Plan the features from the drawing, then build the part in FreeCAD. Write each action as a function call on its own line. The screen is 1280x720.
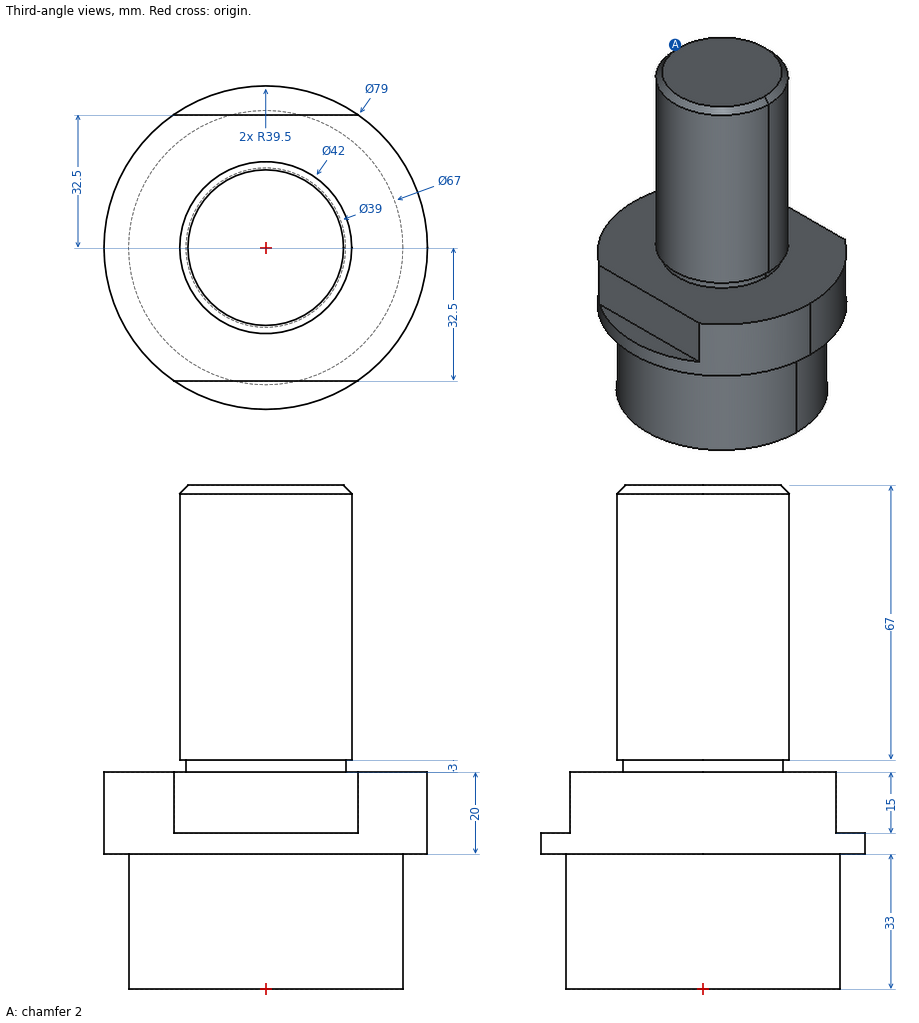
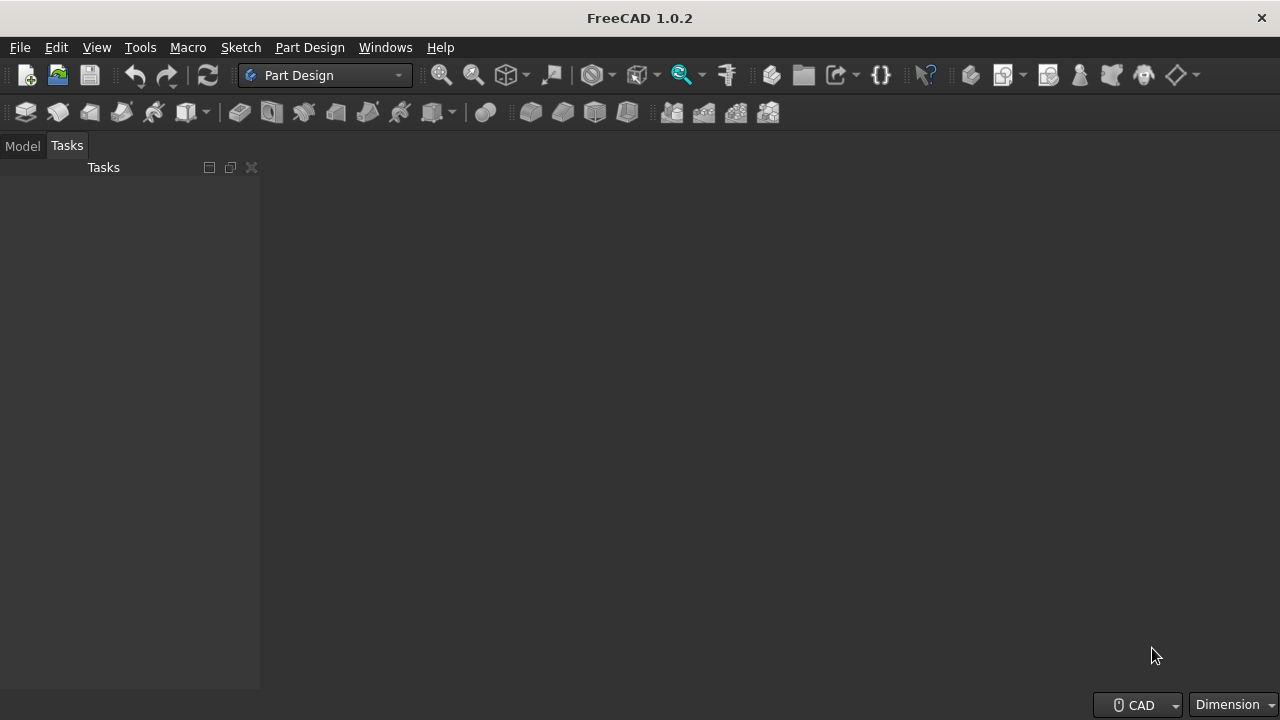
click(26, 76)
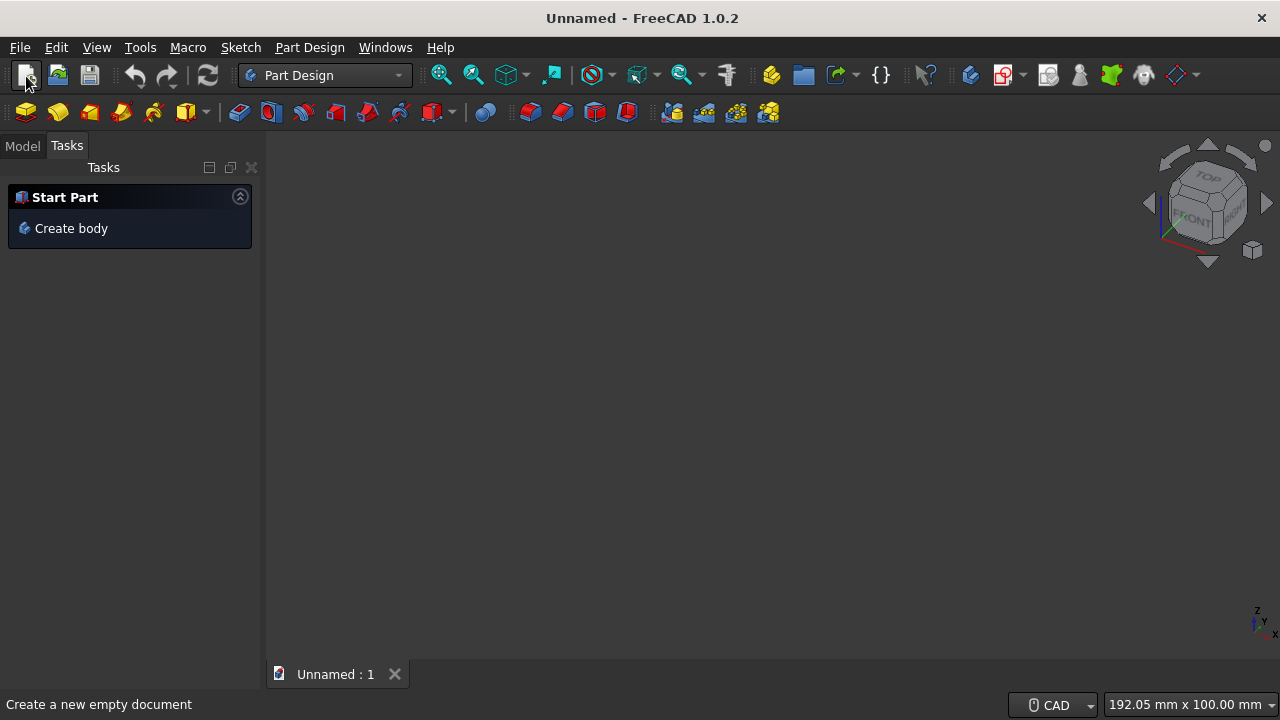
click(1004, 76)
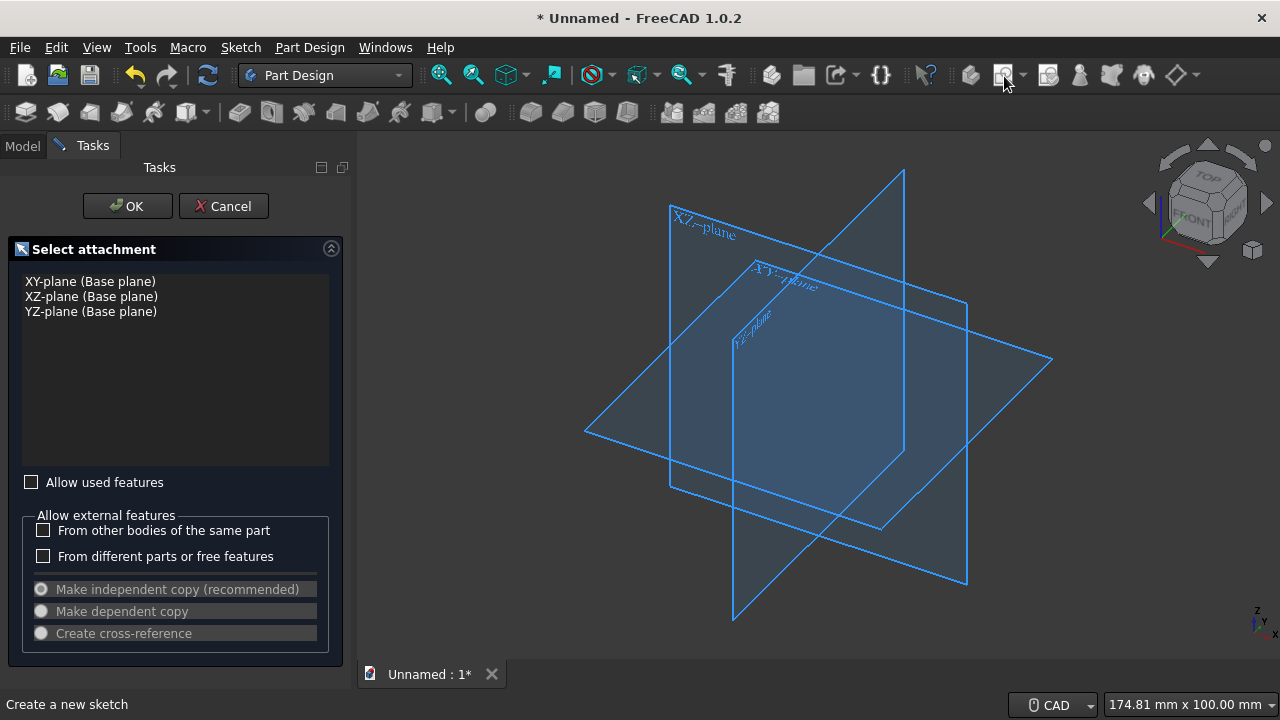
click(82, 282)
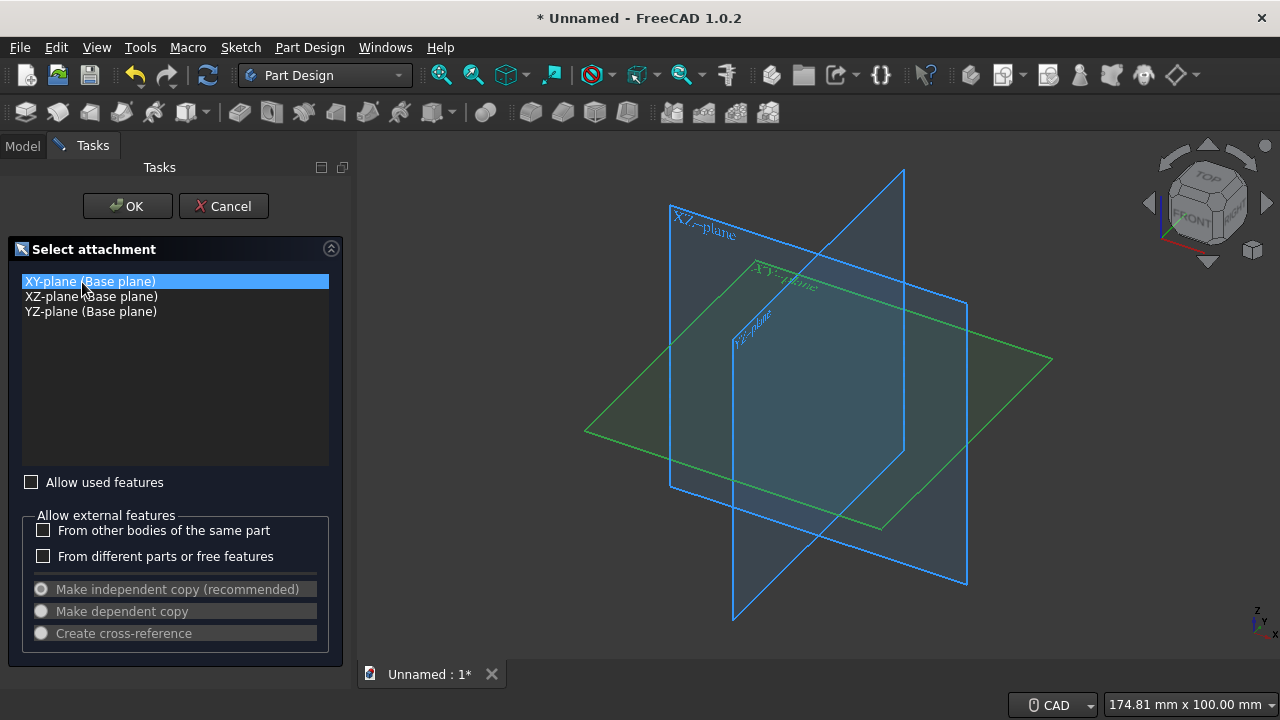
click(128, 206)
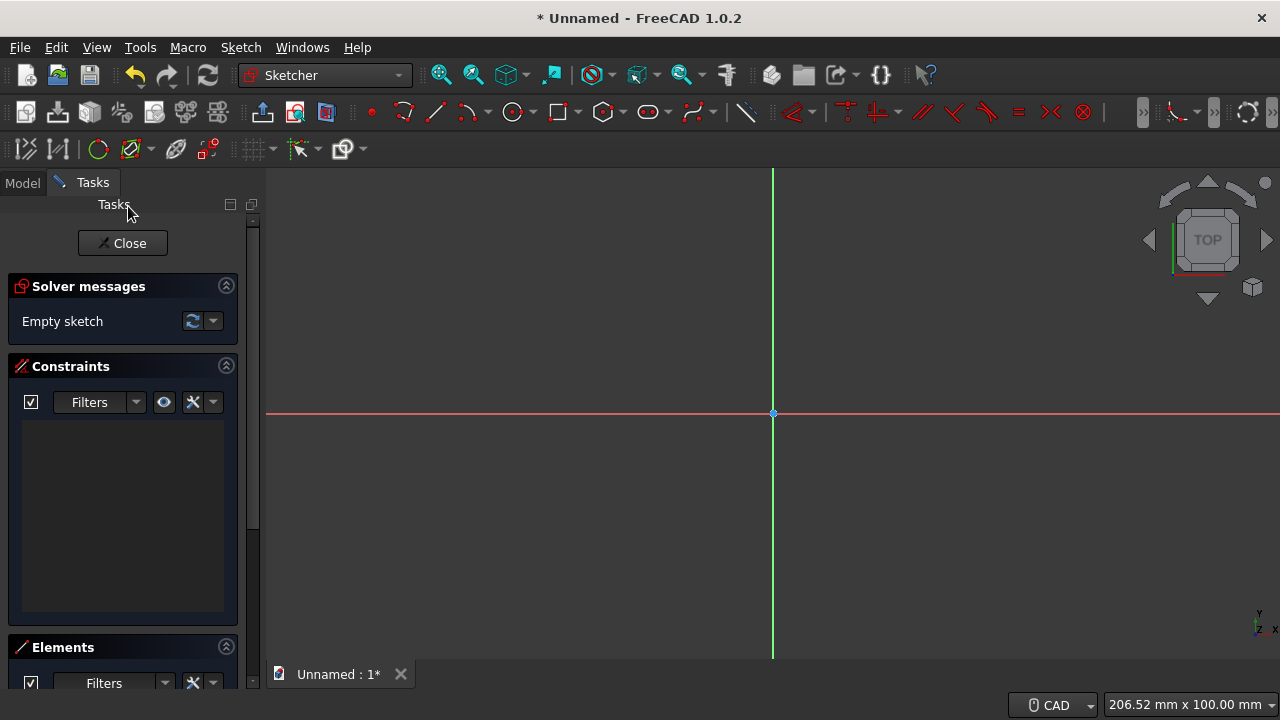
click(514, 112)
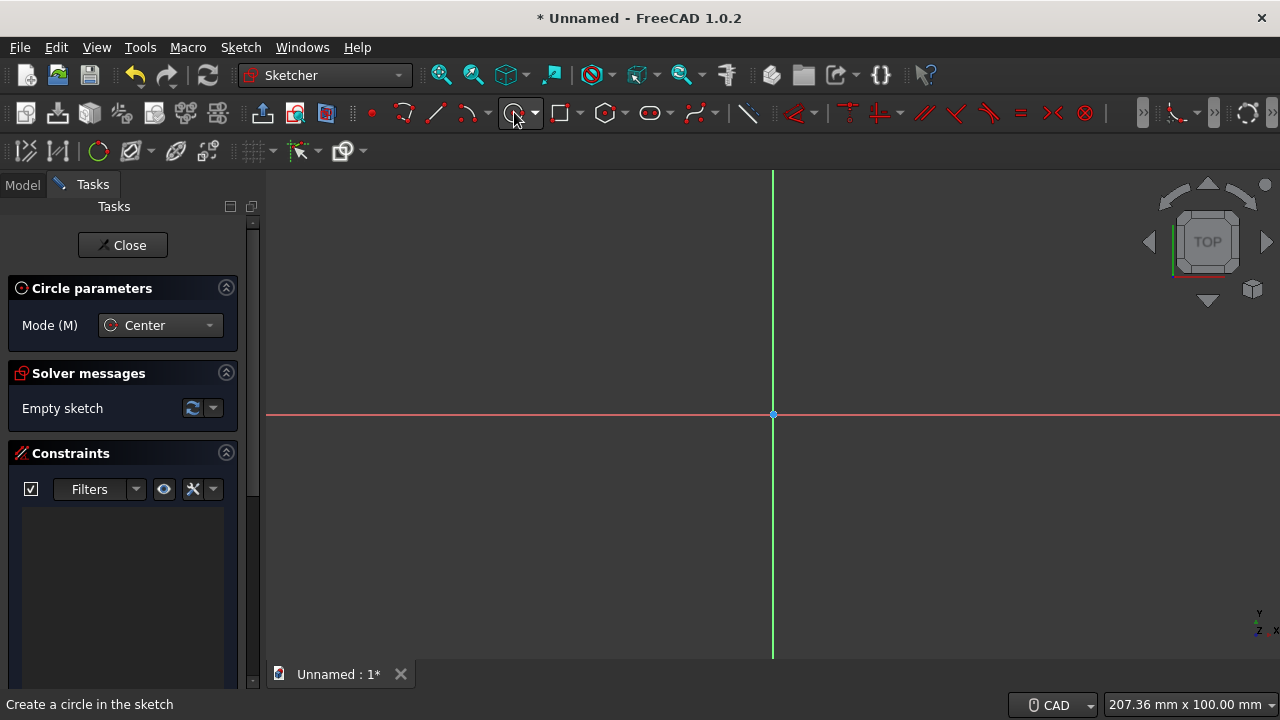
click(773, 414)
move(889, 299)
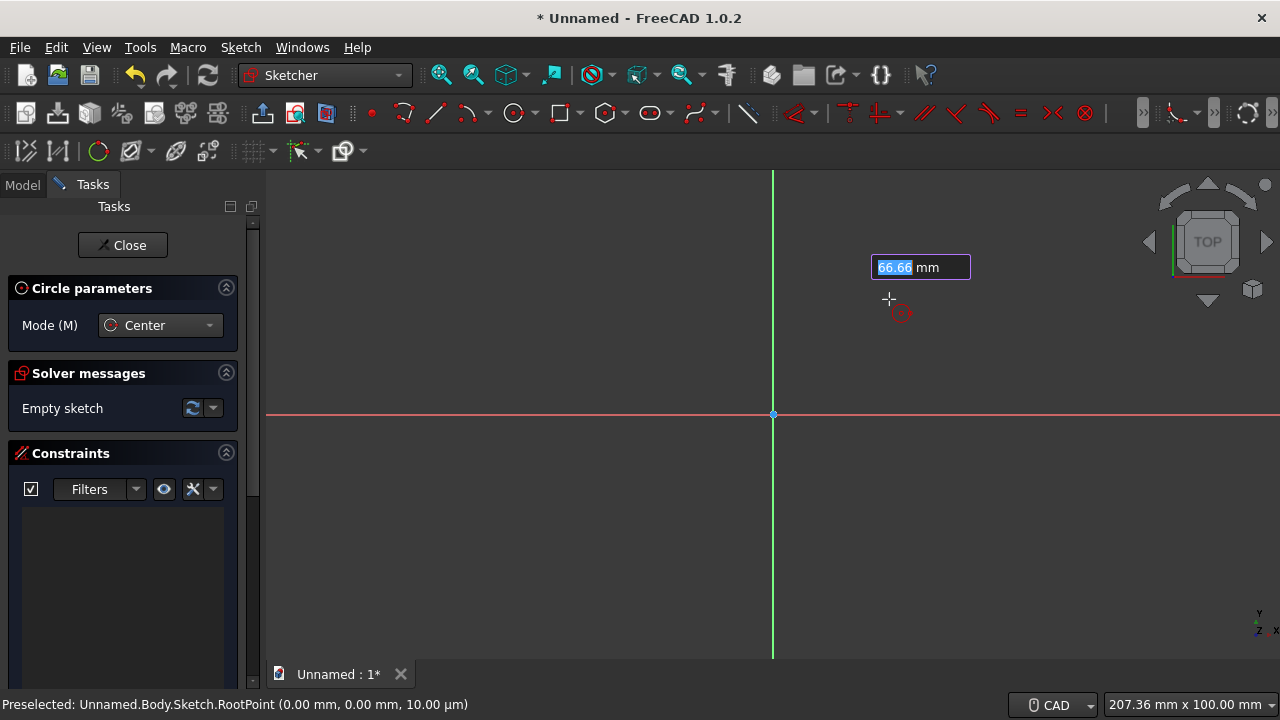
text(67)
key(Return)
key(Escape)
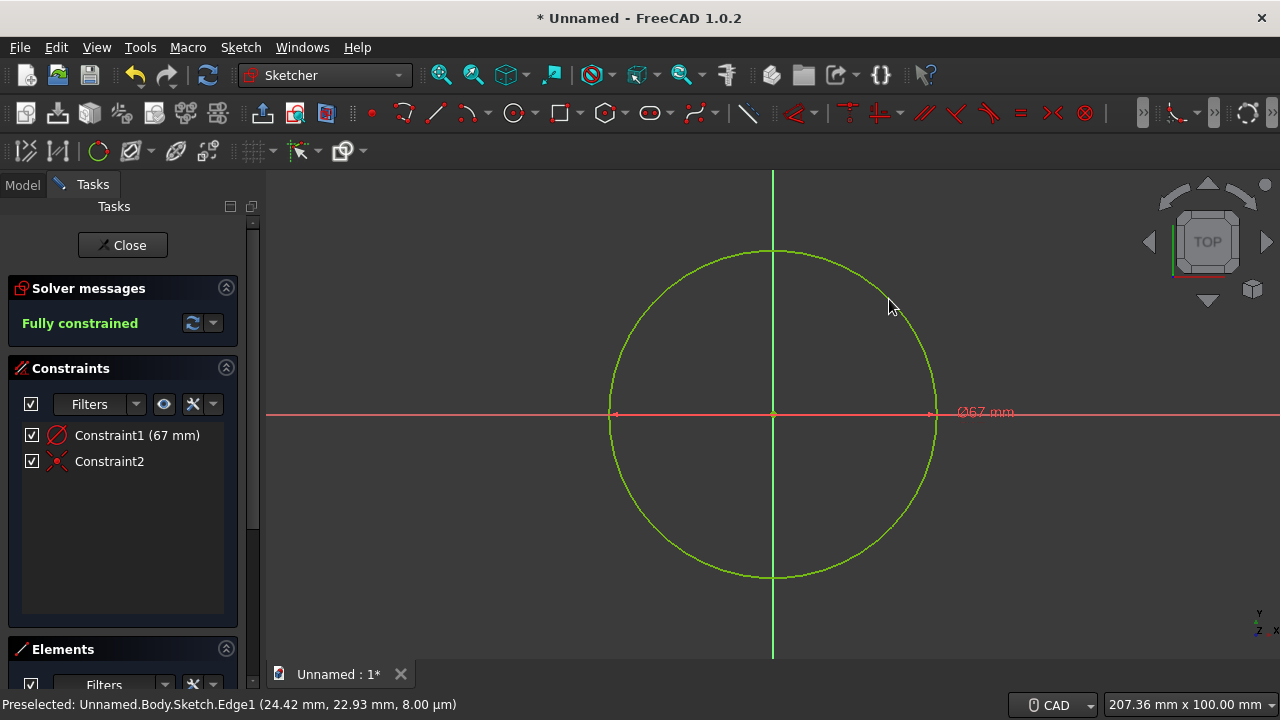
click(123, 245)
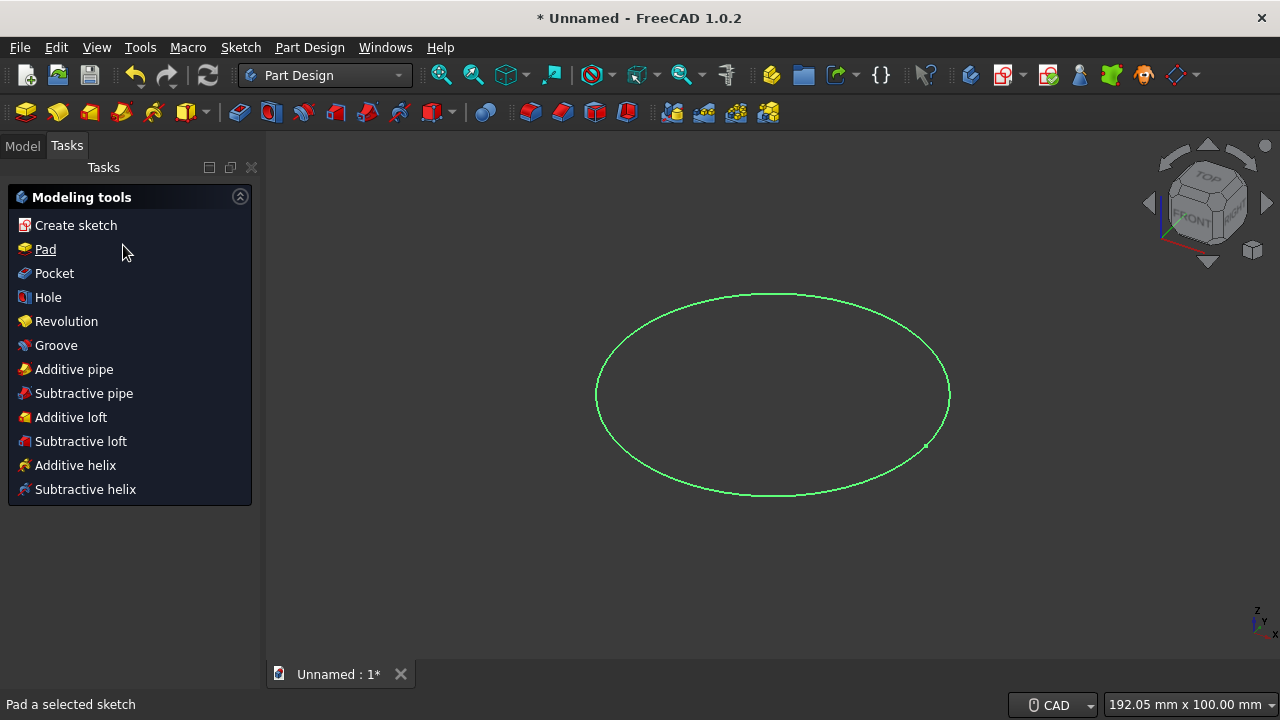
click(26, 112)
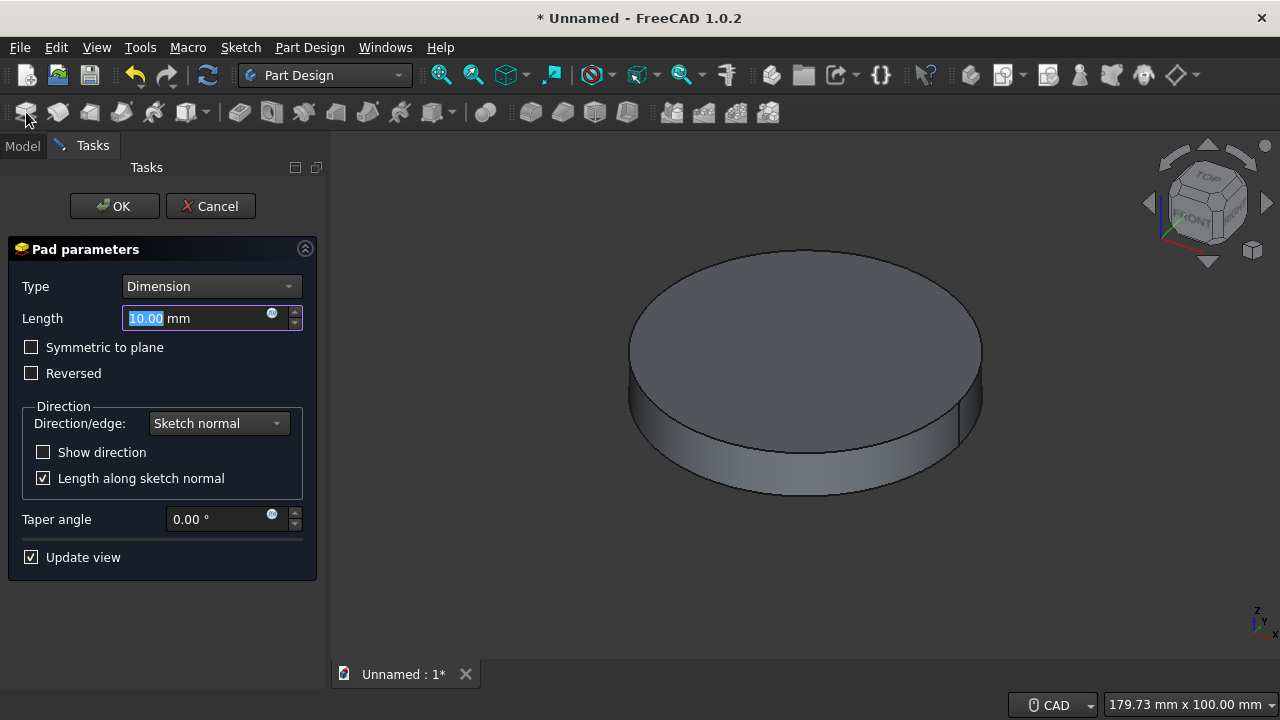
text(33)
key(Tab)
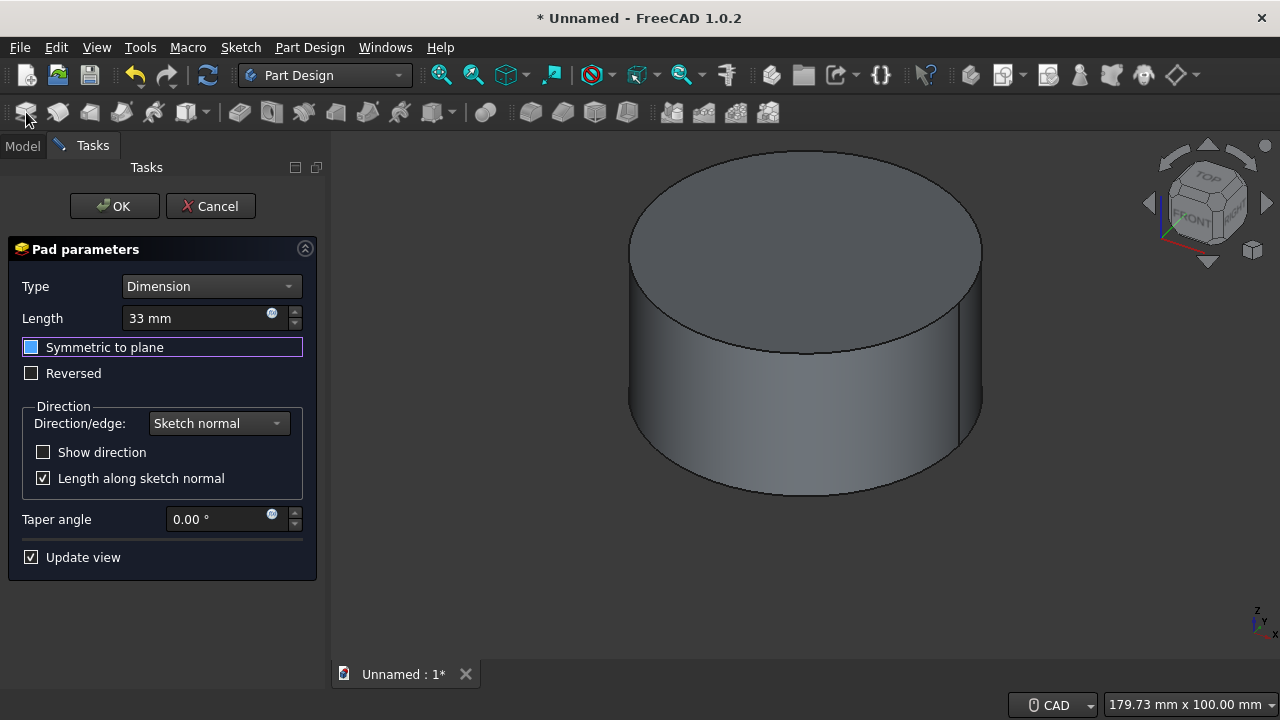
click(115, 206)